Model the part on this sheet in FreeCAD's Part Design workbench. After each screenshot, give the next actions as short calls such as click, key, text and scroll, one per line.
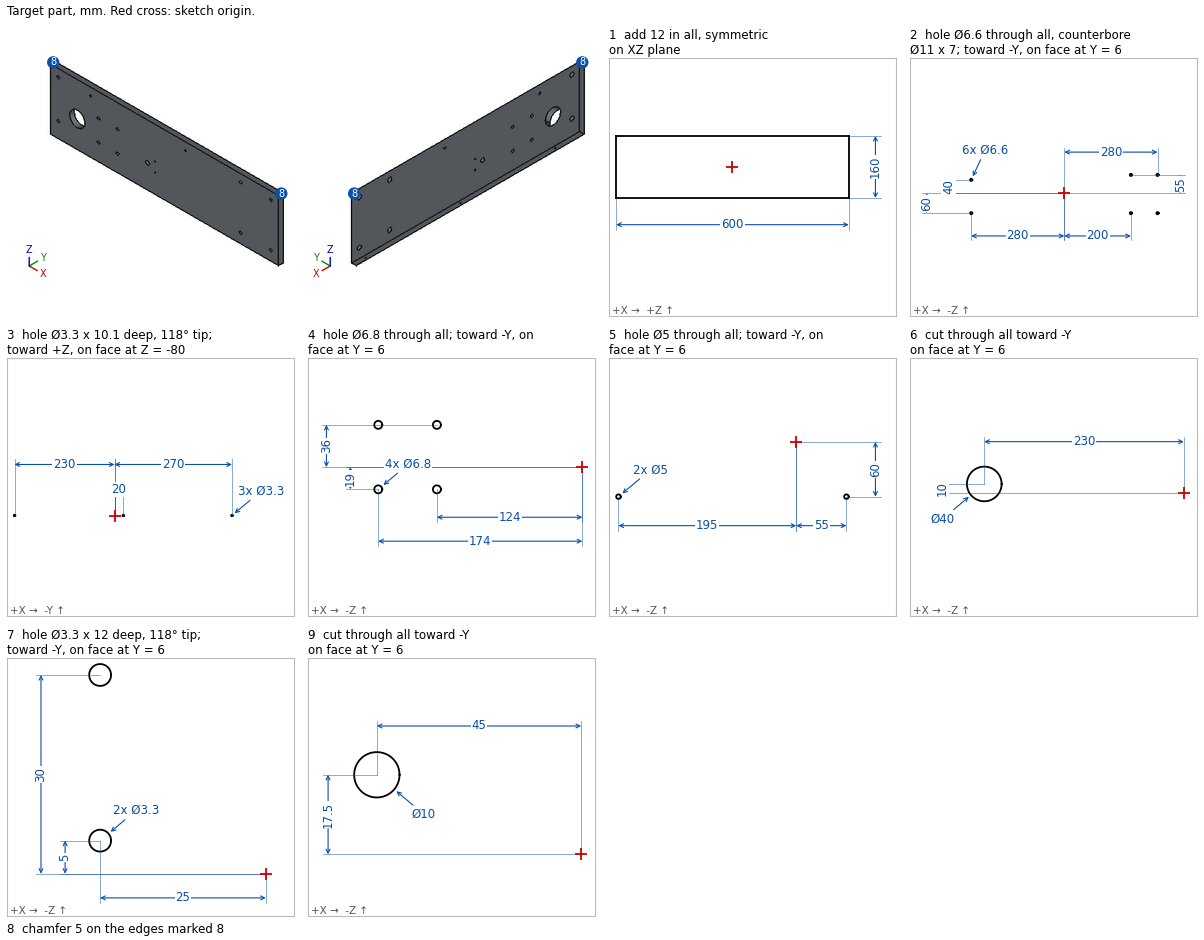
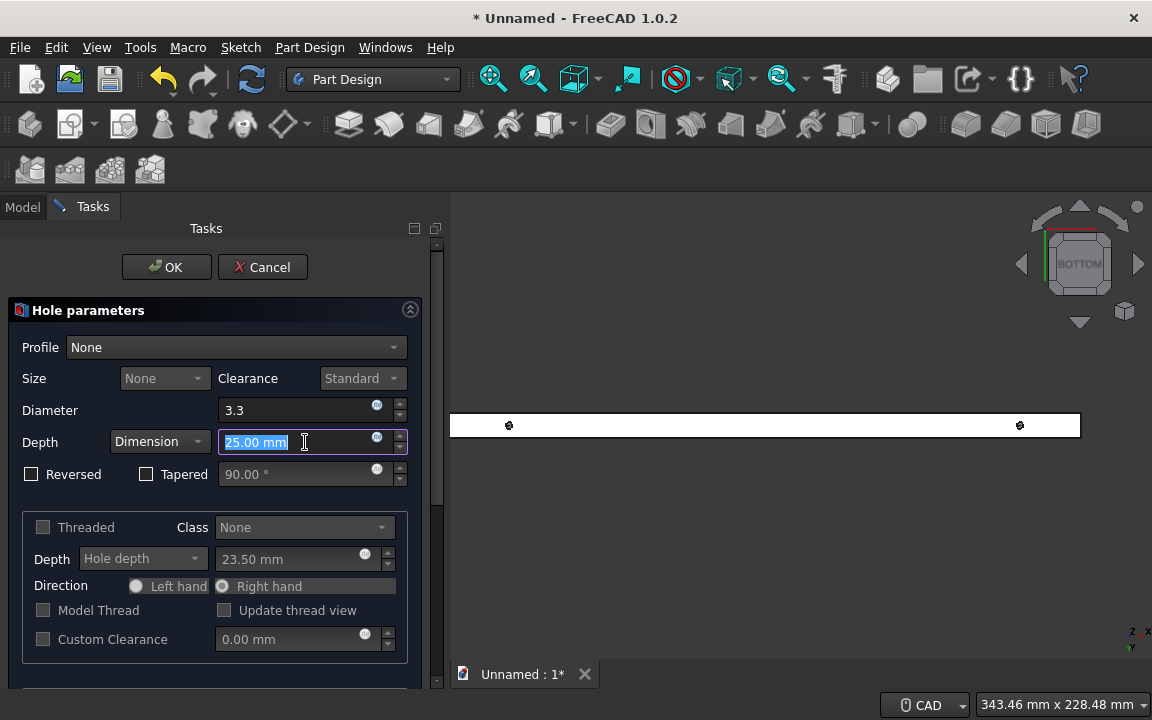
text(10.1)
key(Tab)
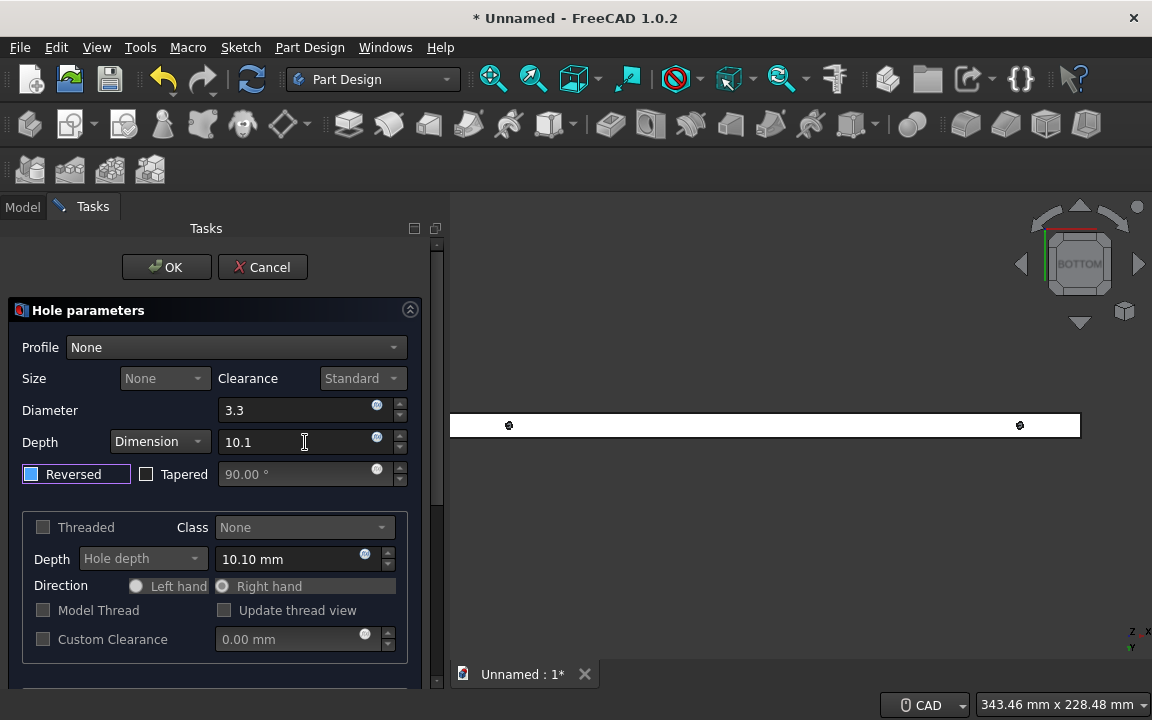
click(167, 267)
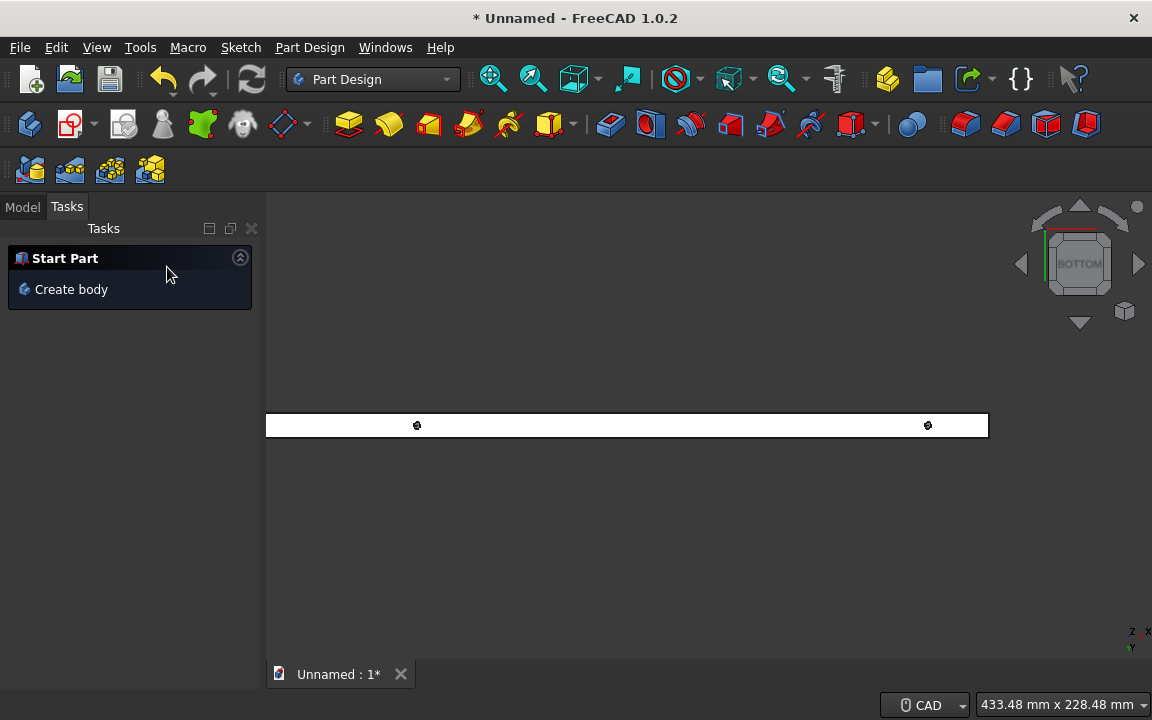
key(v)
key(f)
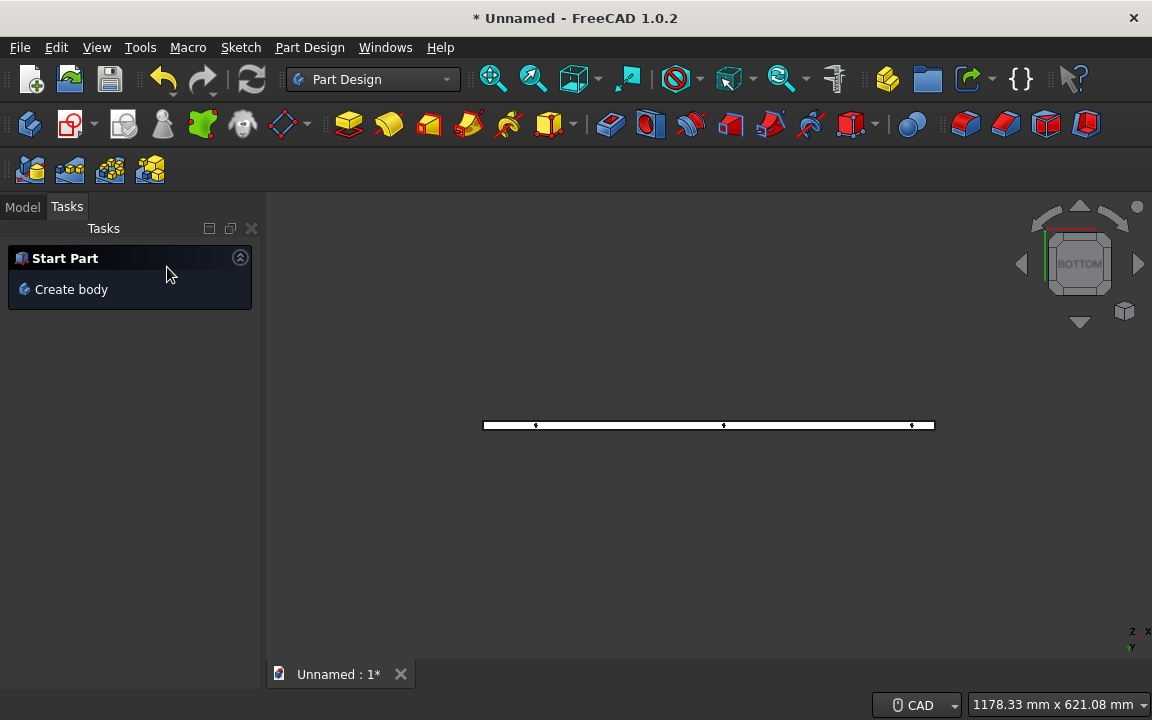
key(4)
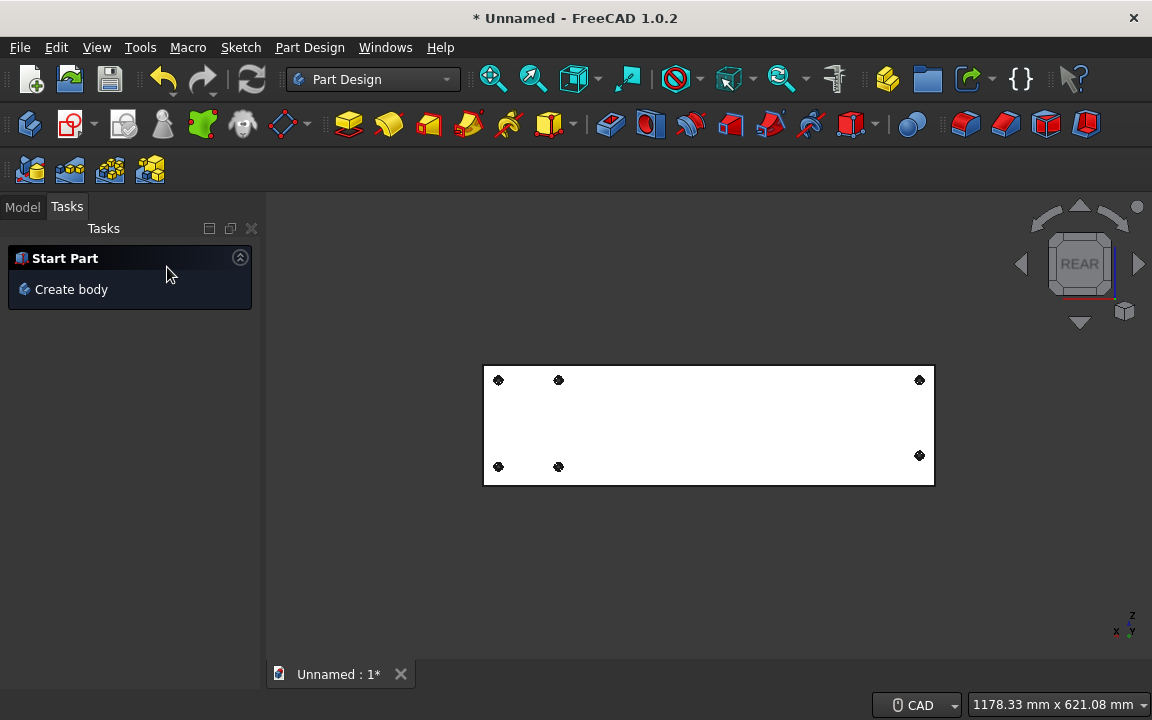
click(645, 424)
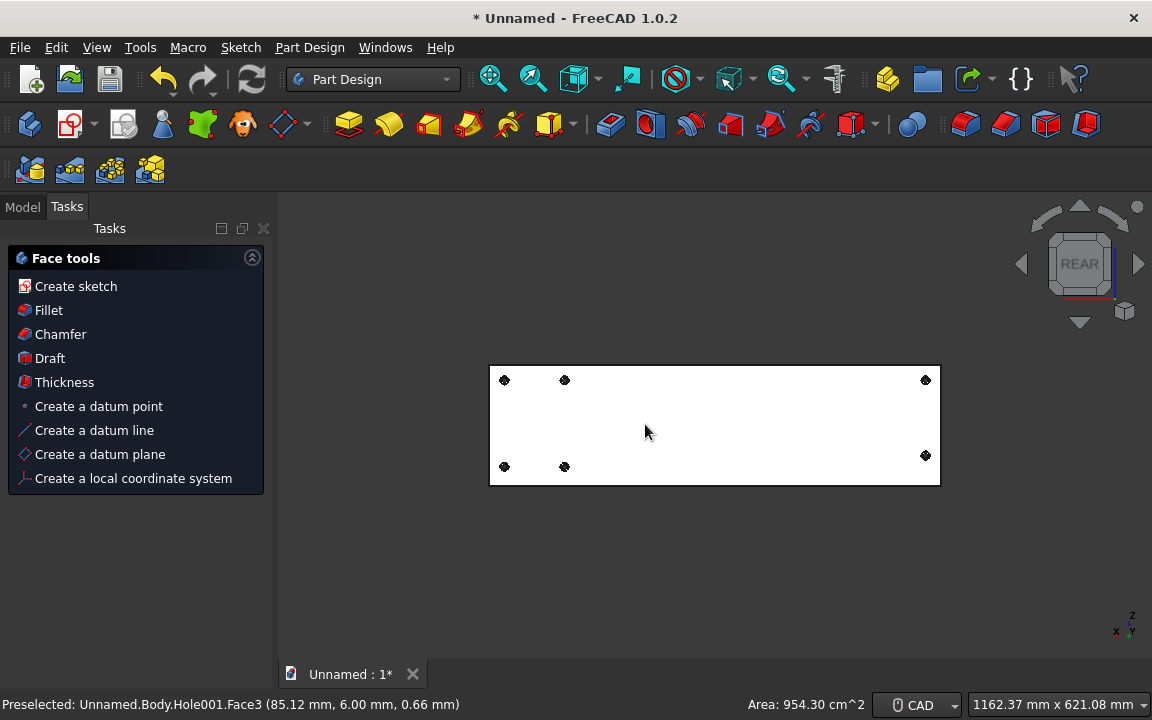
click(70, 124)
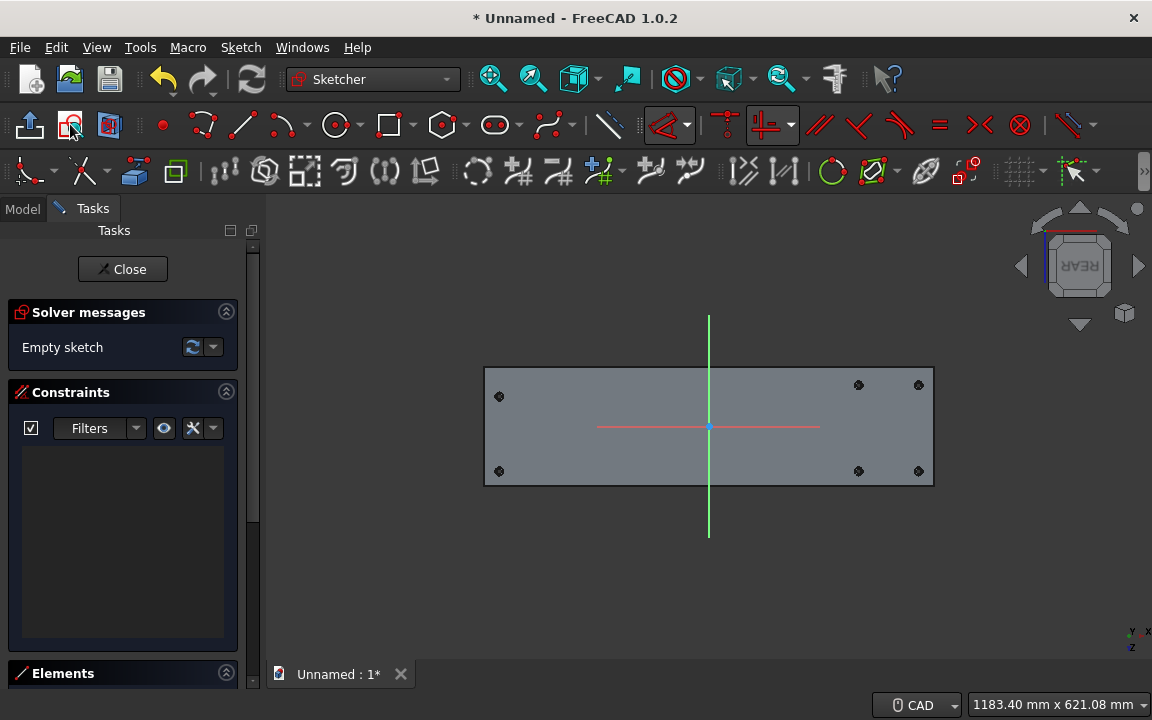
scroll(589, 419, up, 9)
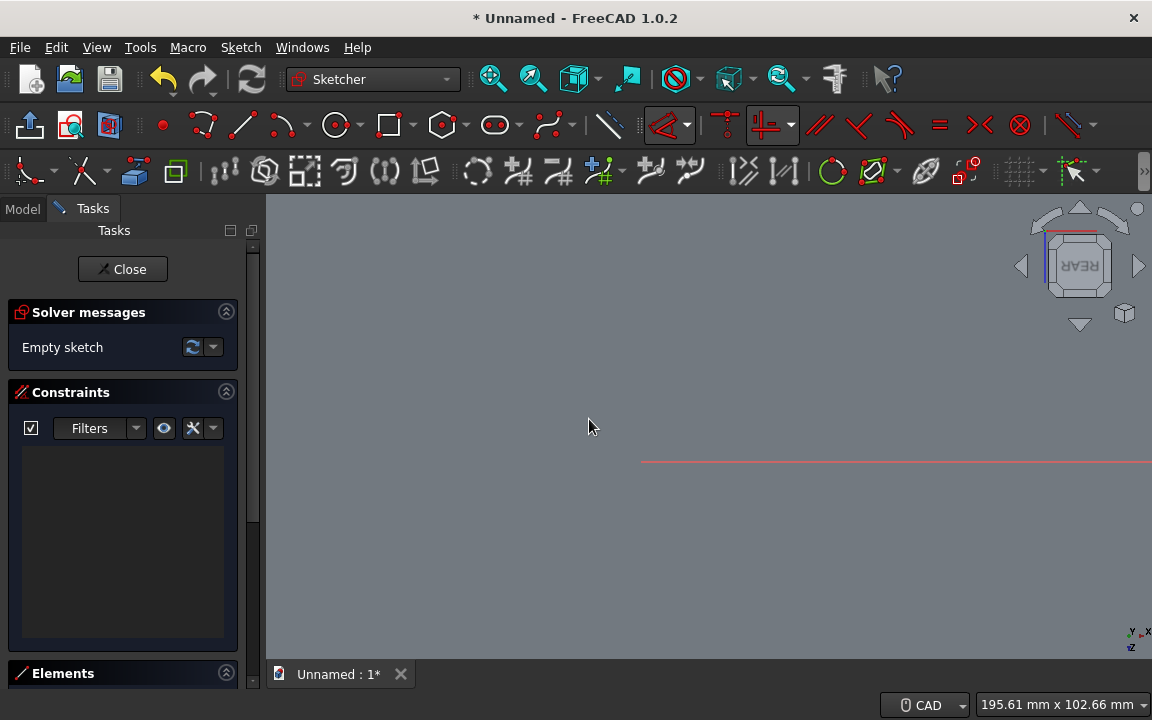
click(336, 126)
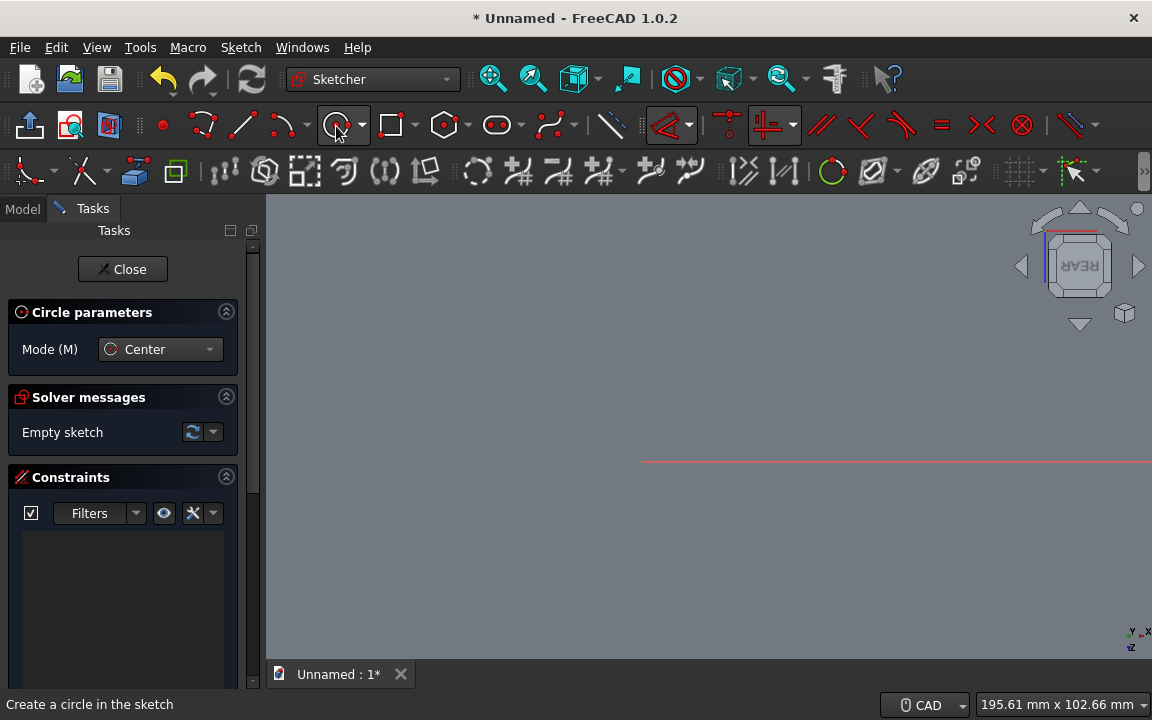
scroll(525, 548, up, 2)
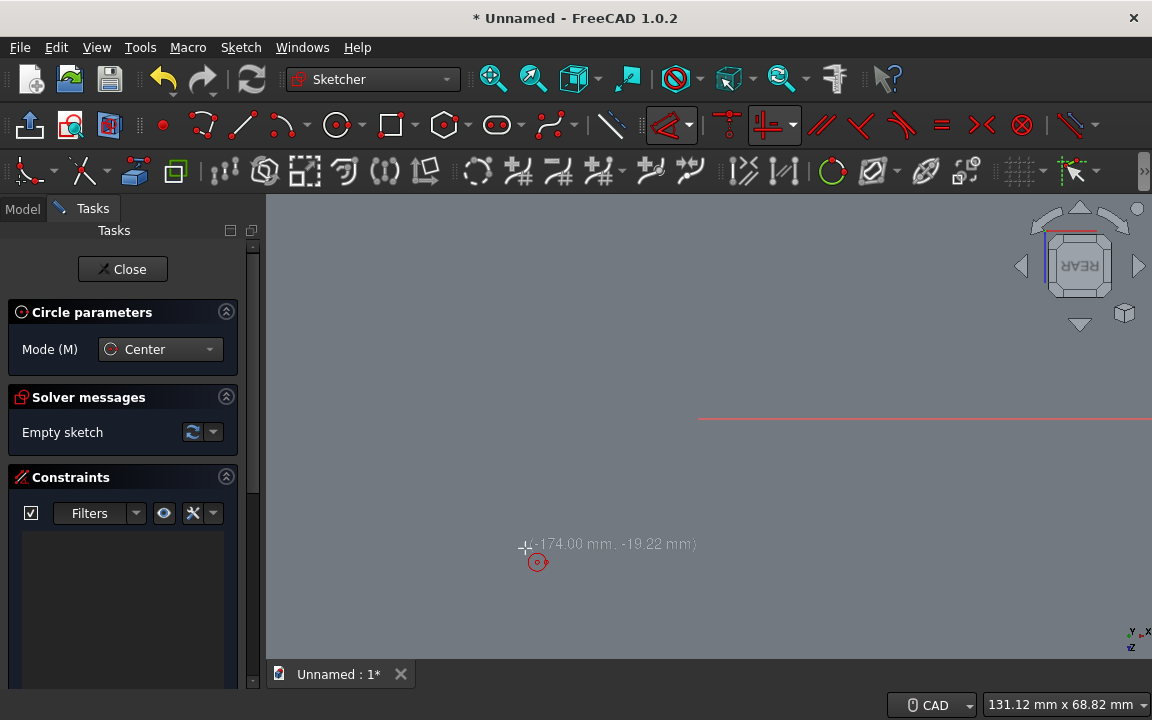
click(525, 548)
move(541, 531)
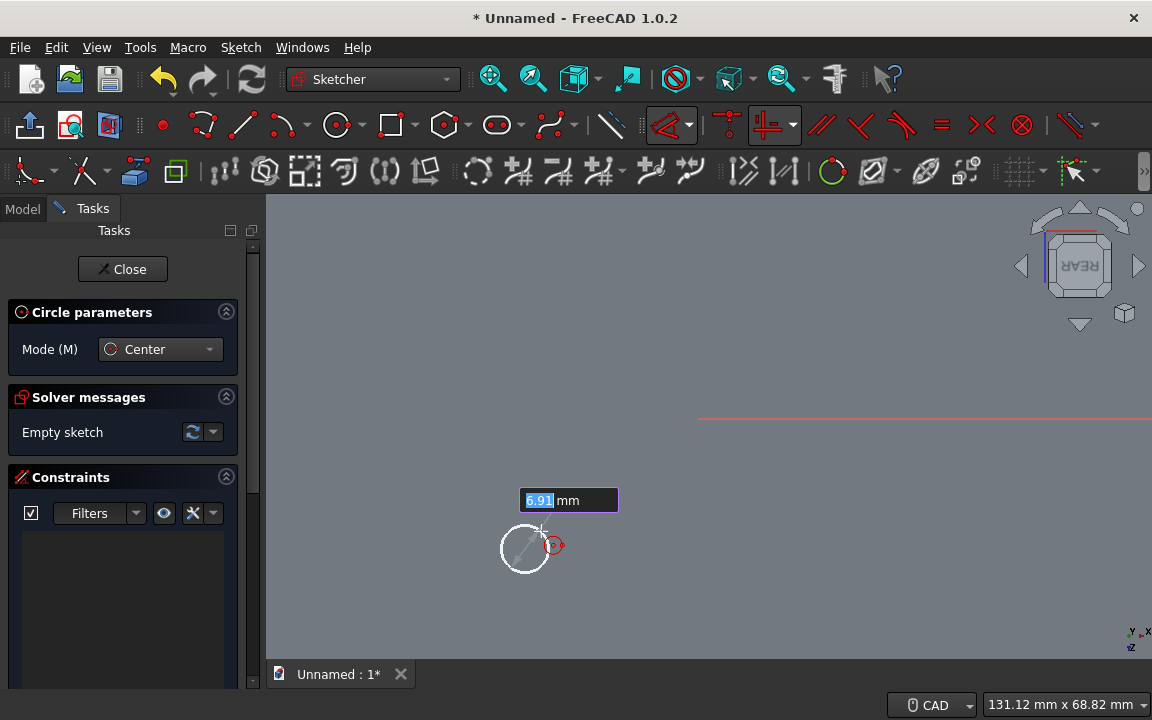
text(6.8)
key(Return)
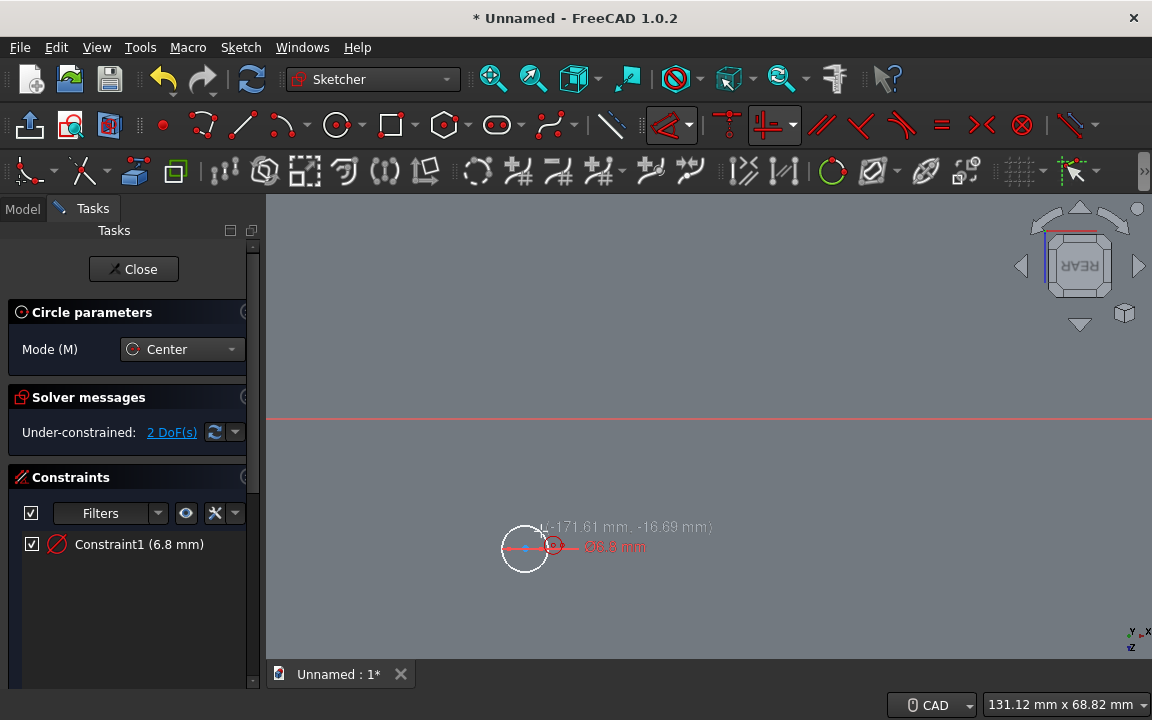
click(863, 548)
move(879, 531)